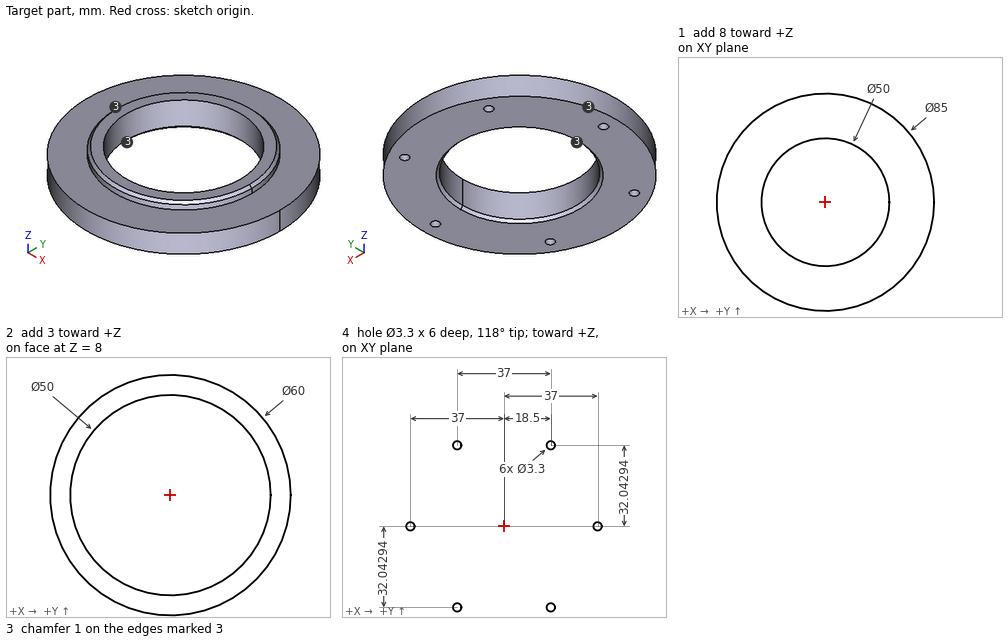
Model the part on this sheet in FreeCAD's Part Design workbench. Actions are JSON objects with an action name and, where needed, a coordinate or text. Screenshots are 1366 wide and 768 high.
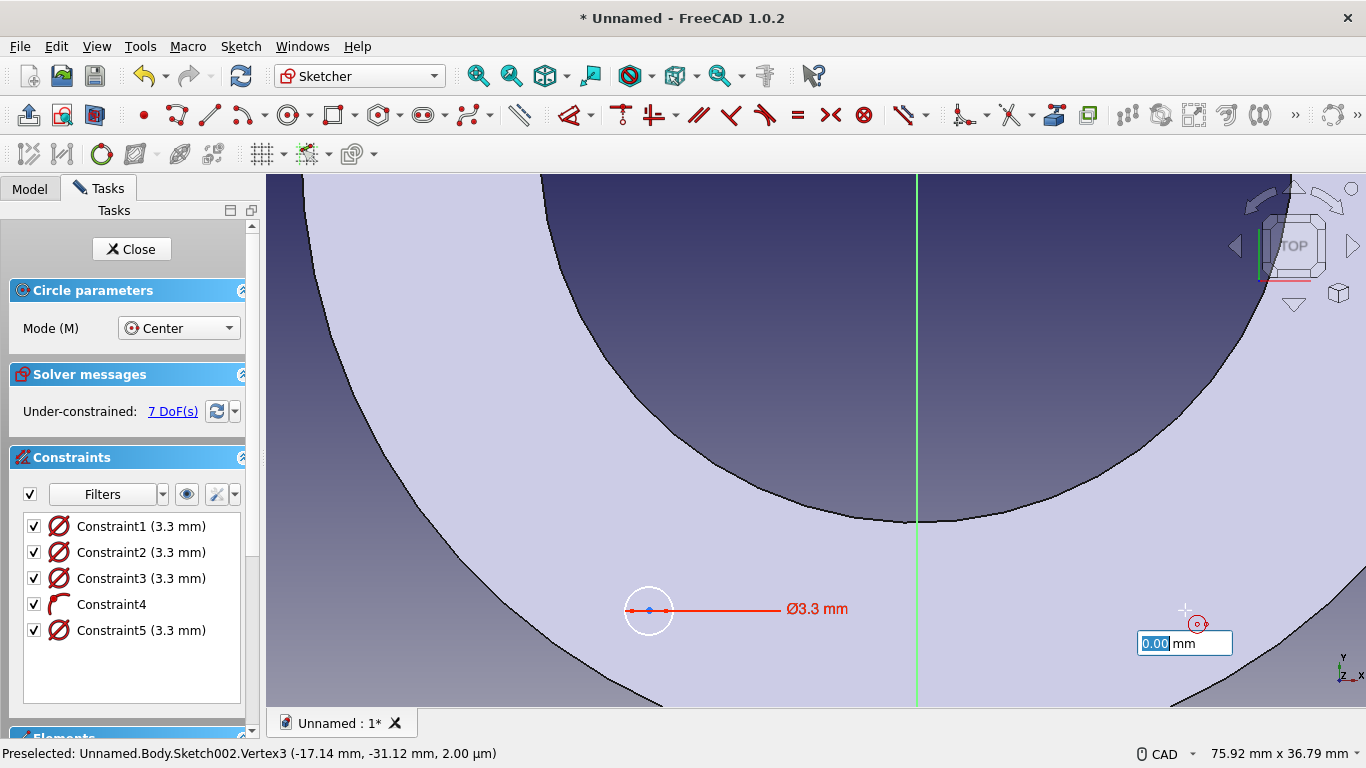
{"action": "scroll", "coordinate": [649, 612], "scroll_direction": "down", "scroll_amount": 5}
{"action": "mouse_move", "coordinate": [852, 606]}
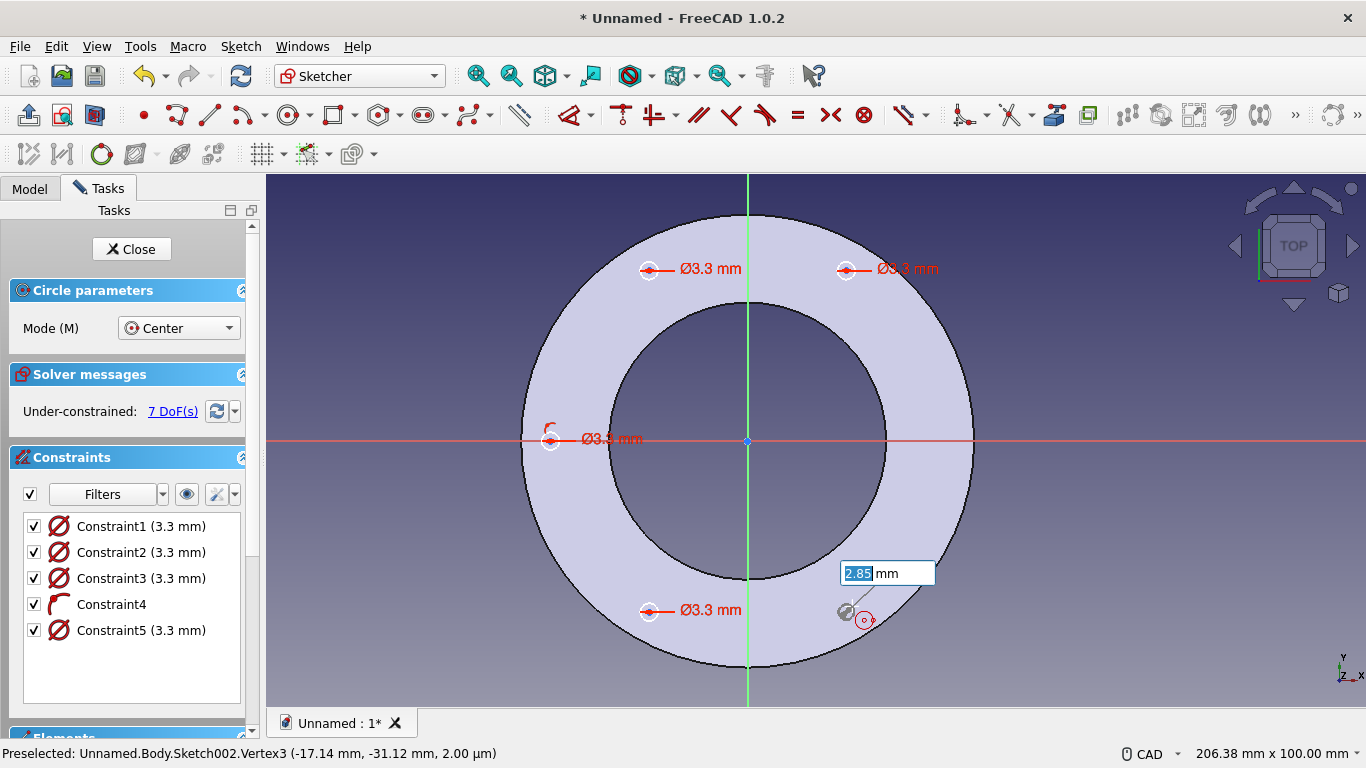
{"action": "type", "text": "3.3"}
{"action": "key", "text": "Return"}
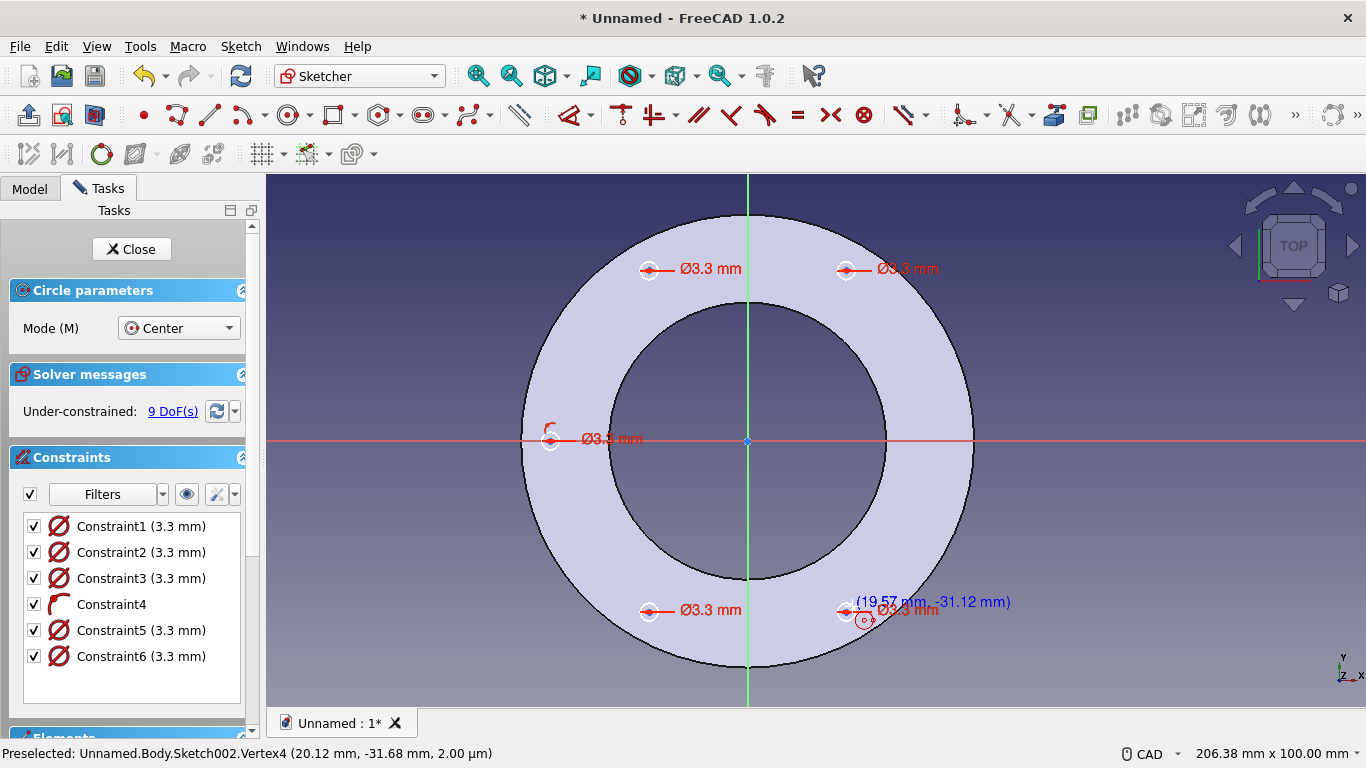
{"action": "scroll", "coordinate": [945, 441], "scroll_direction": "up", "scroll_amount": 5}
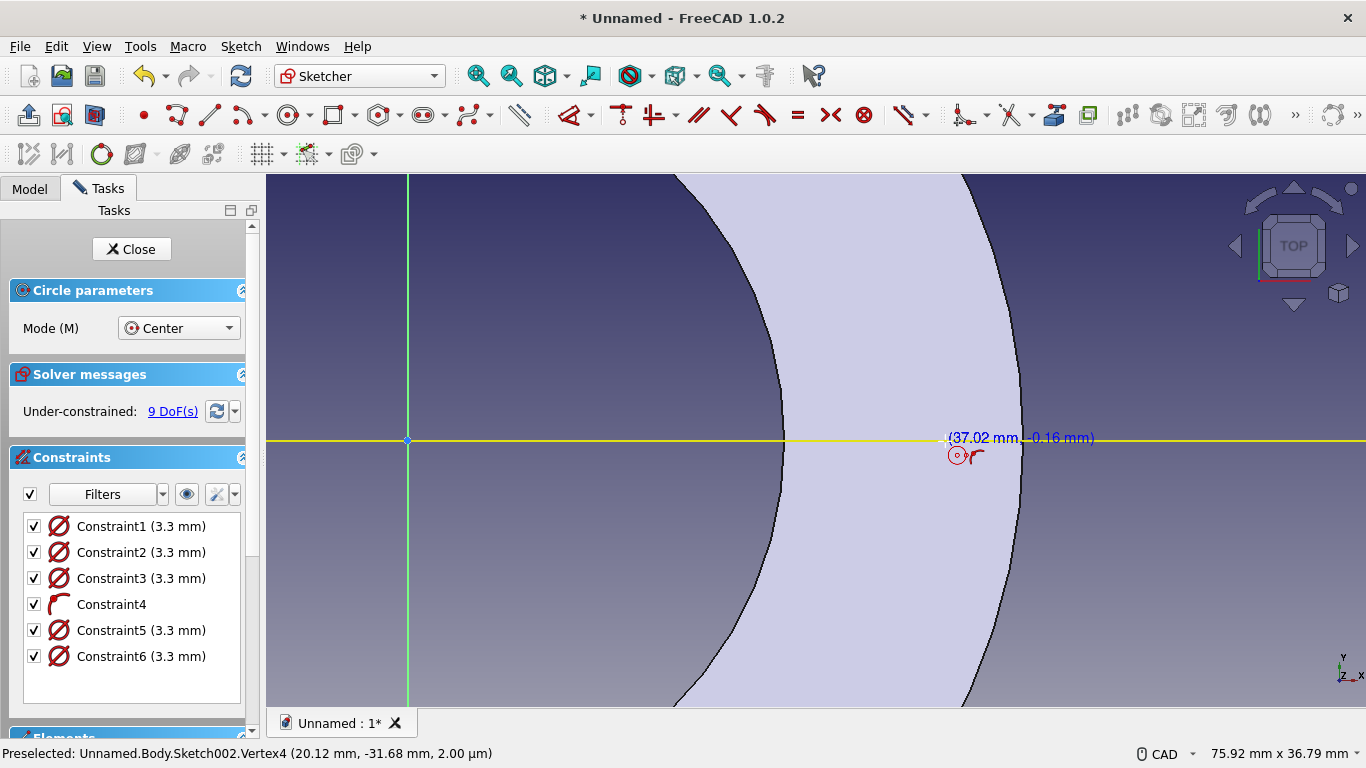
{"action": "left_click", "coordinate": [944, 440]}
{"action": "mouse_move", "coordinate": [961, 424]}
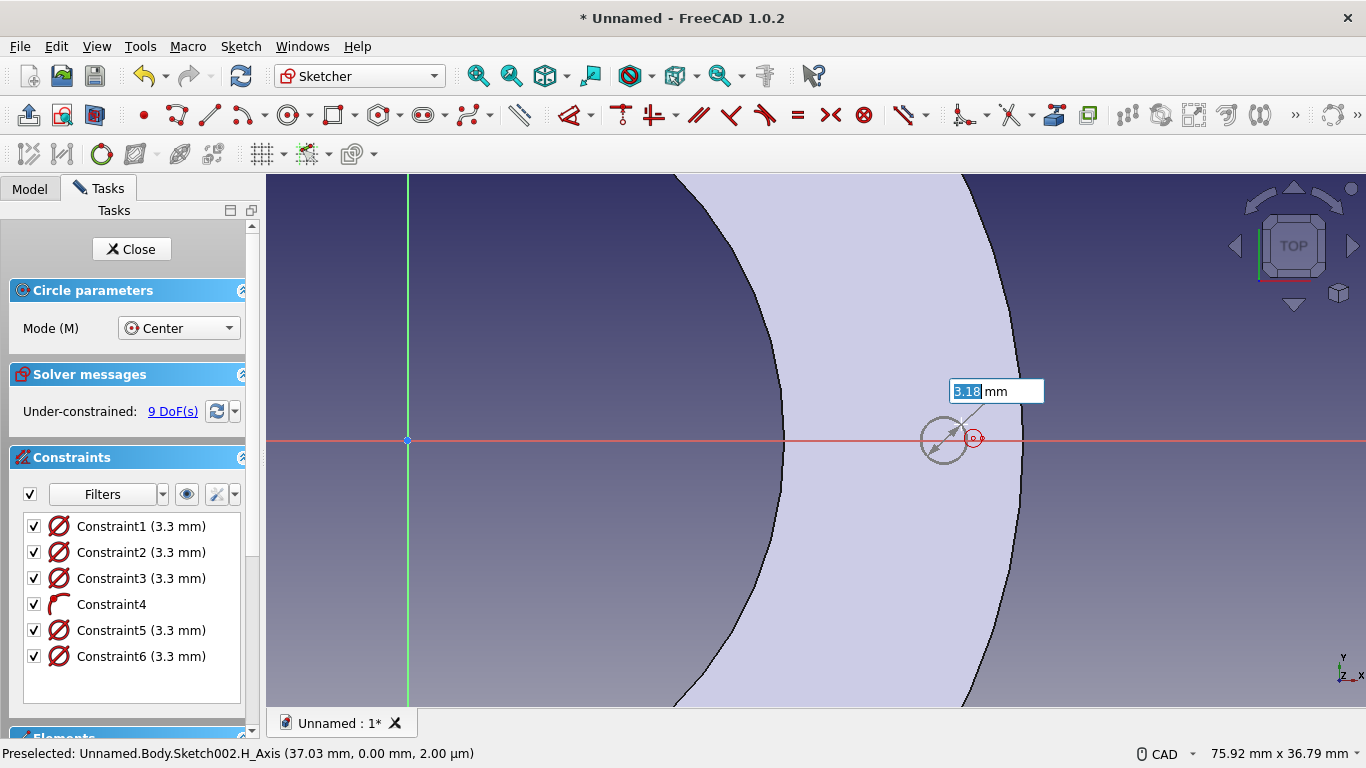
{"action": "type", "text": "3.3"}
{"action": "key", "text": "Return"}
{"action": "key", "text": "Escape"}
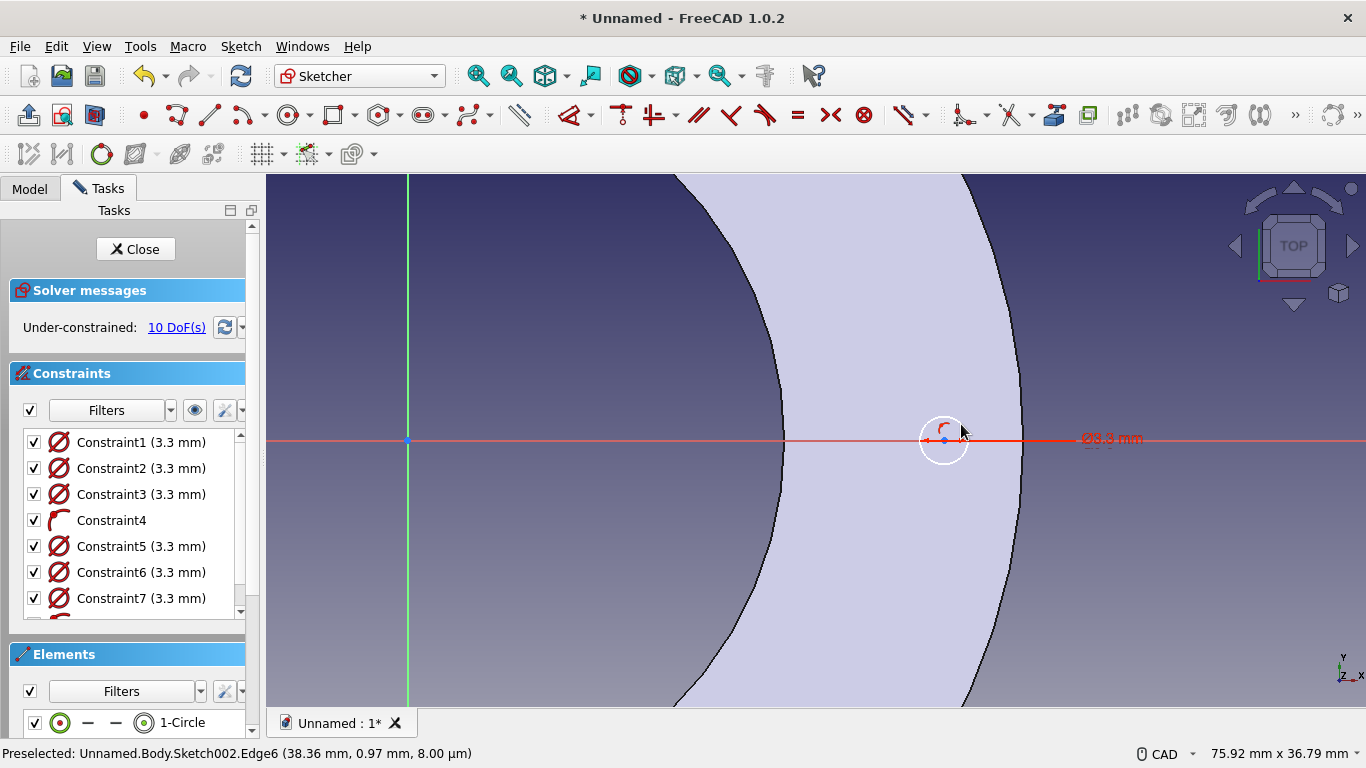
{"action": "scroll", "coordinate": [945, 441], "scroll_direction": "down", "scroll_amount": 5}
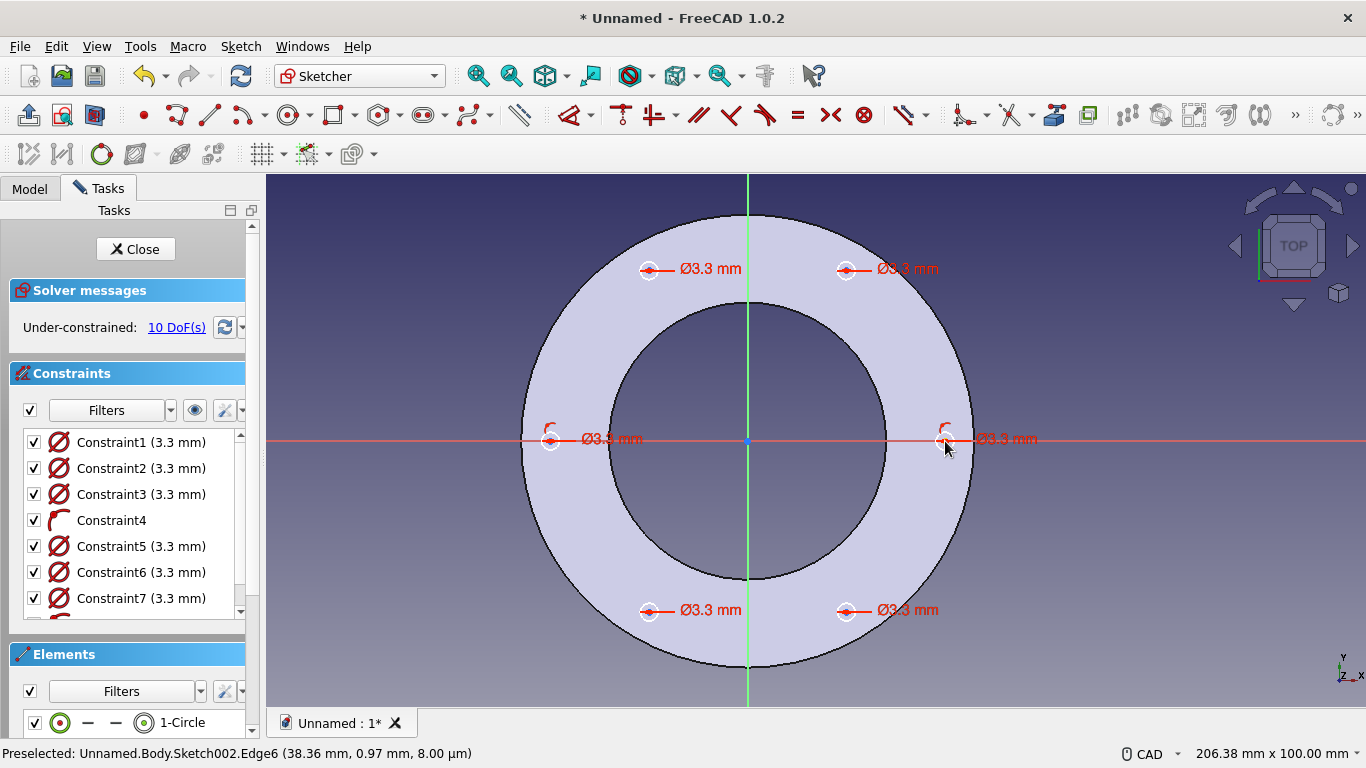
{"action": "left_click", "coordinate": [846, 271]}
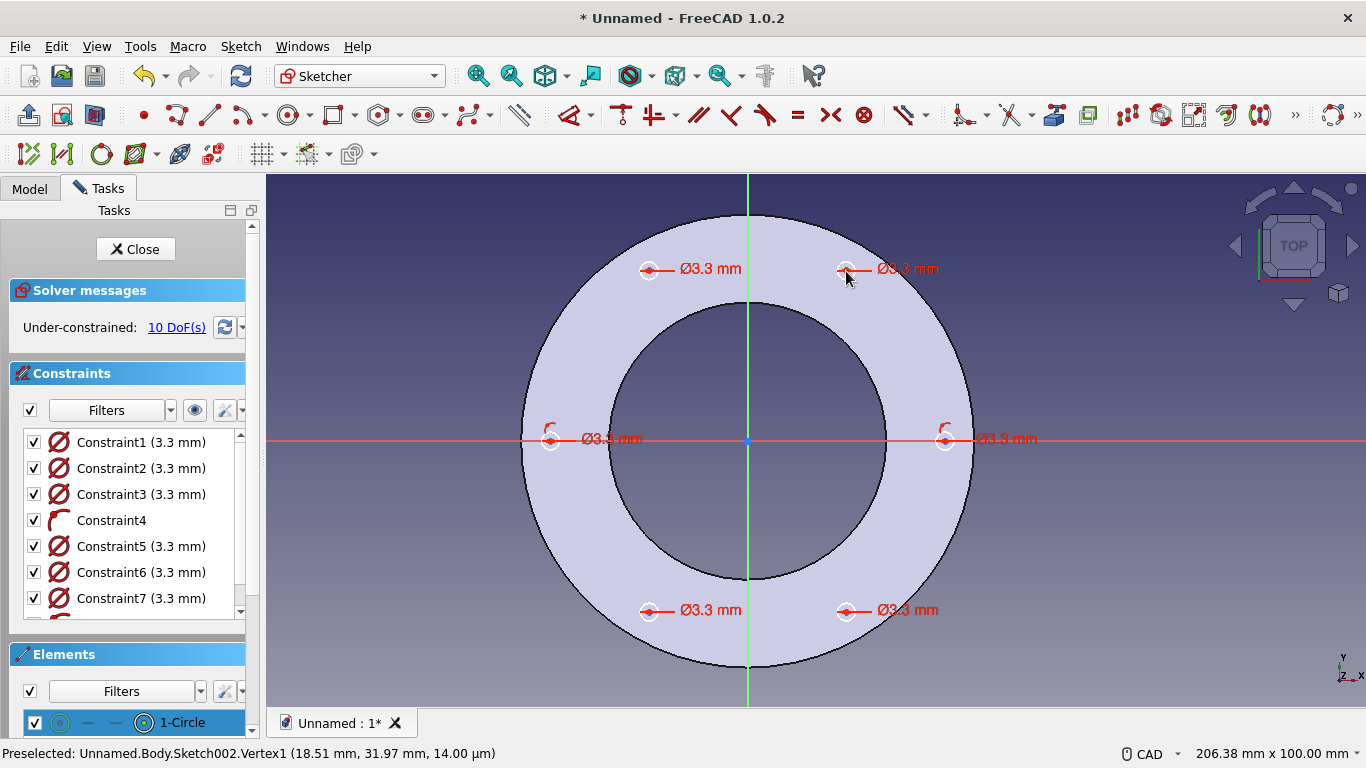
{"action": "left_click", "coordinate": [649, 271]}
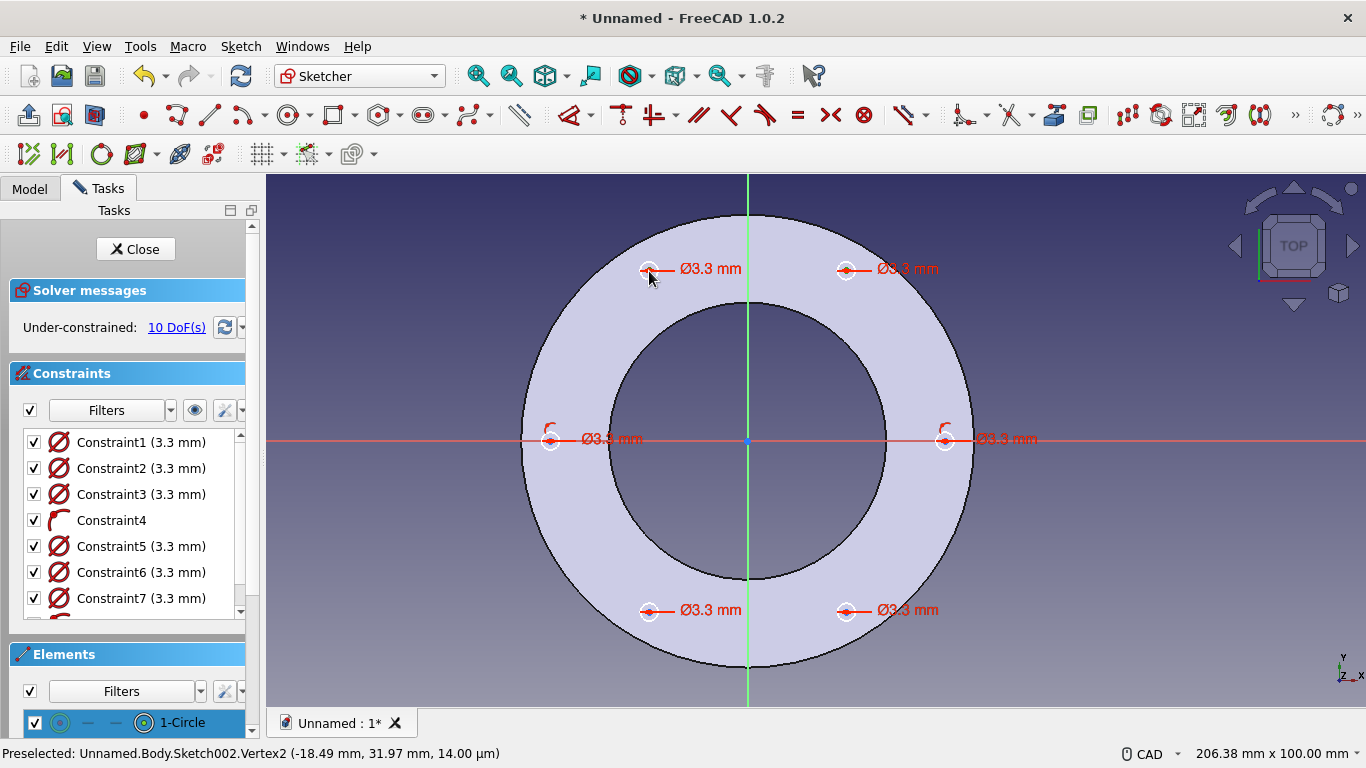
{"action": "left_click", "coordinate": [676, 116]}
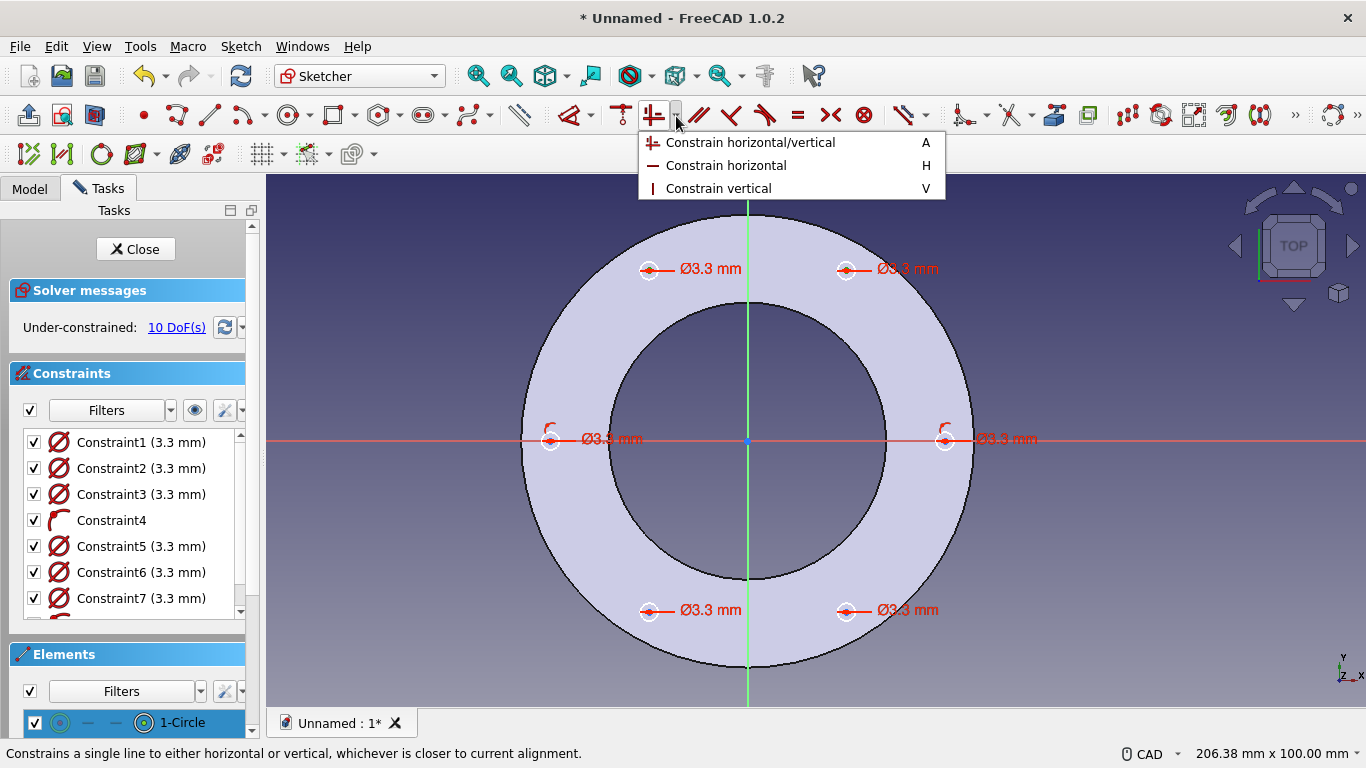
{"action": "left_click", "coordinate": [792, 166]}